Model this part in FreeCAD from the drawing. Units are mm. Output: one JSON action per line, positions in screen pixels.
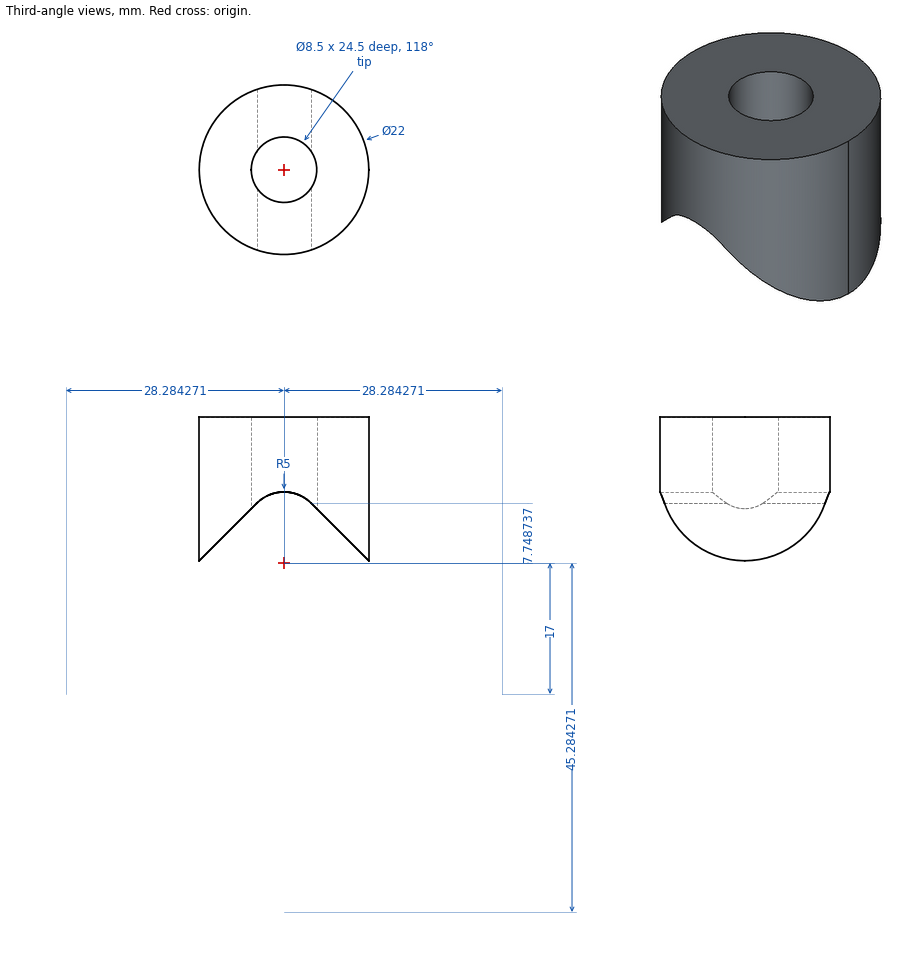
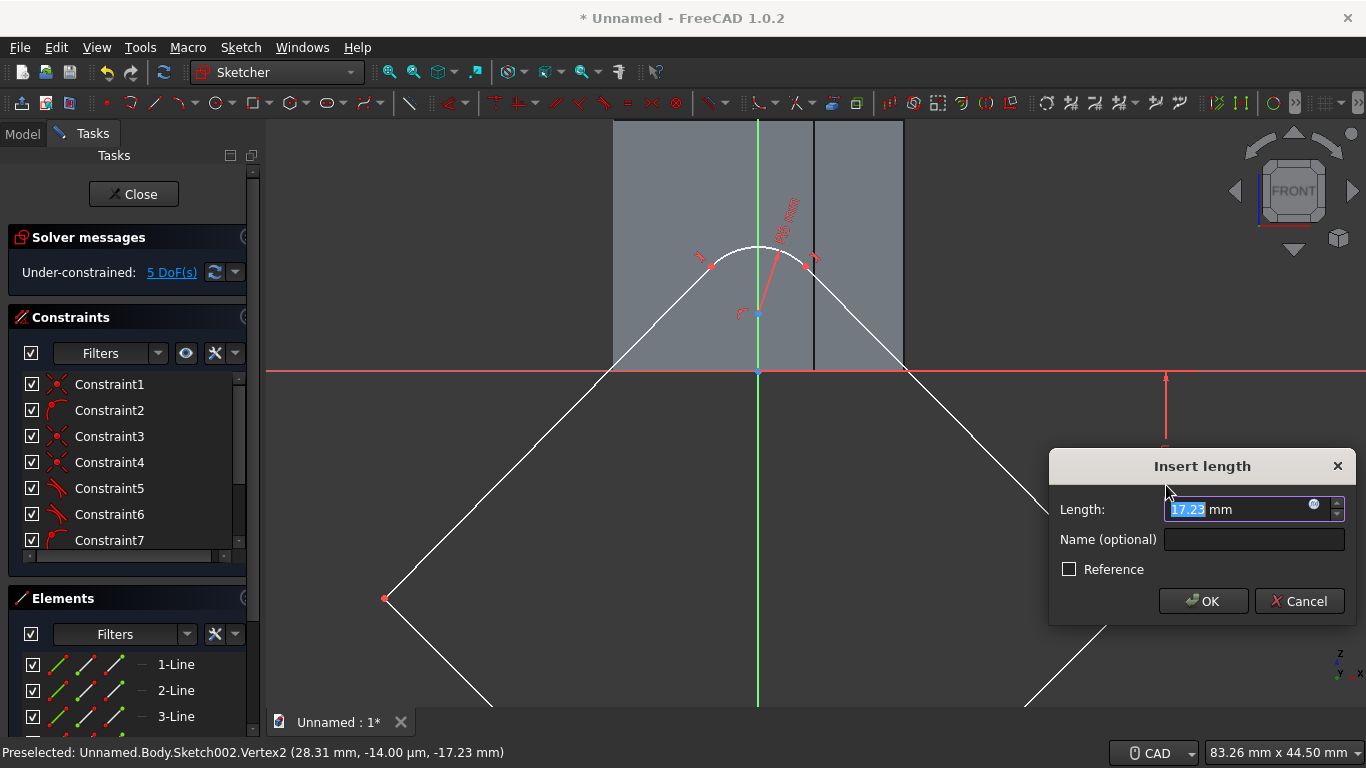
{"action": "type", "text": "17"}
{"action": "key", "text": "Return"}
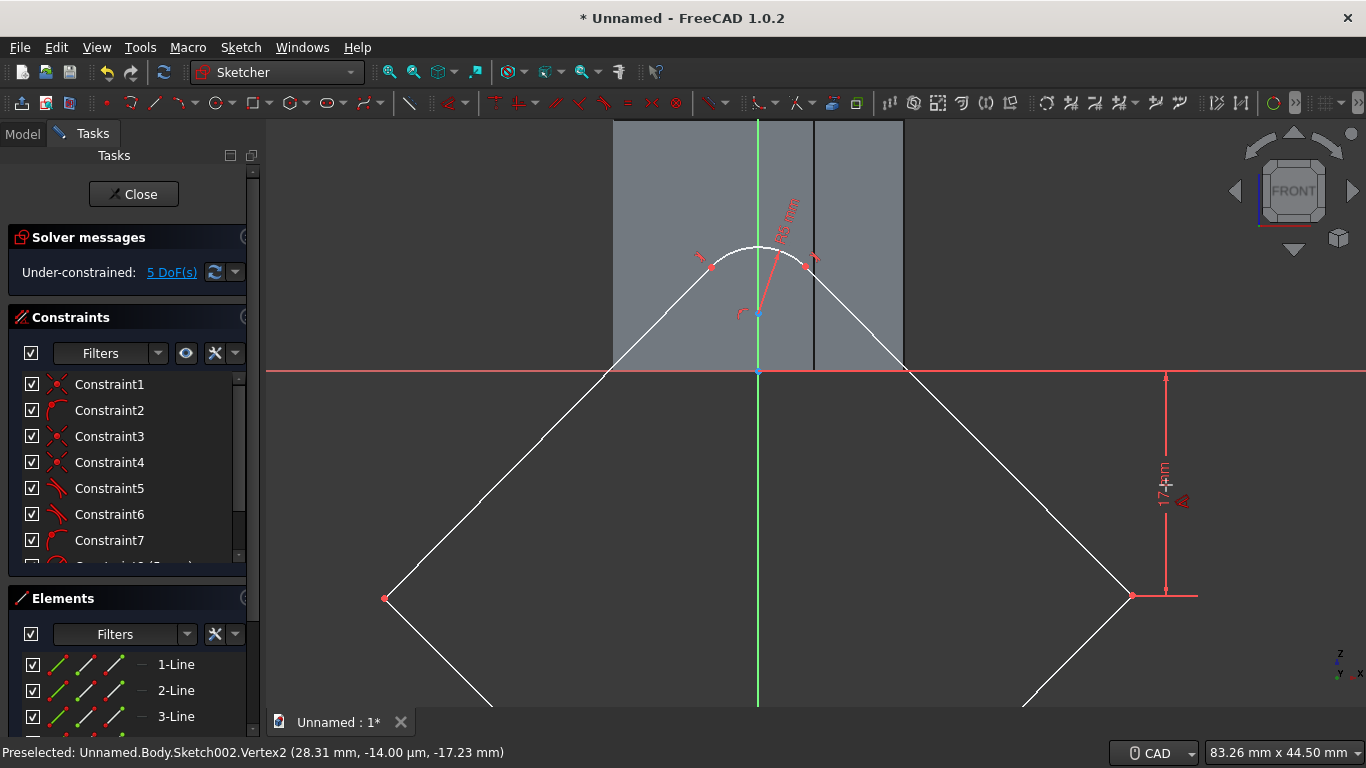
{"action": "left_click", "coordinate": [385, 599]}
{"action": "left_click", "coordinate": [351, 485]}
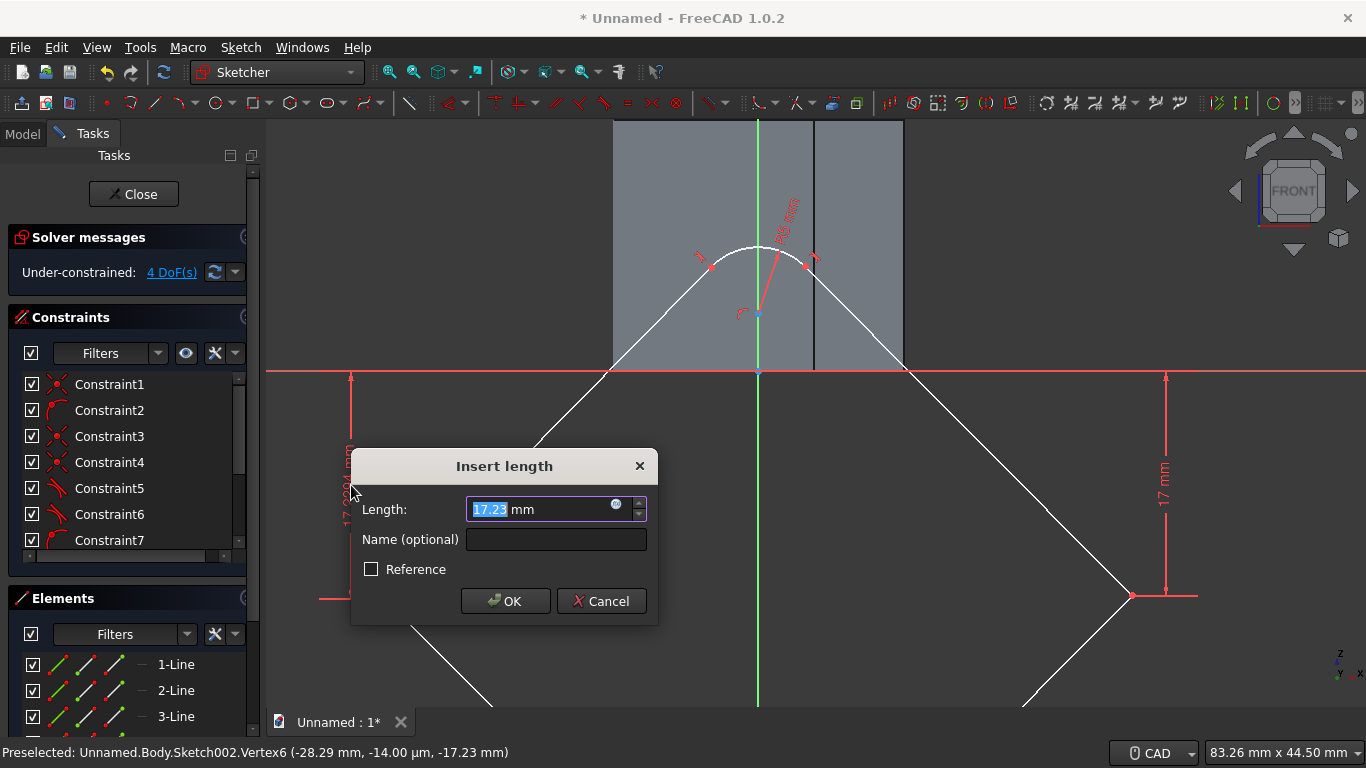
{"action": "type", "text": "17"}
{"action": "key", "text": "Return"}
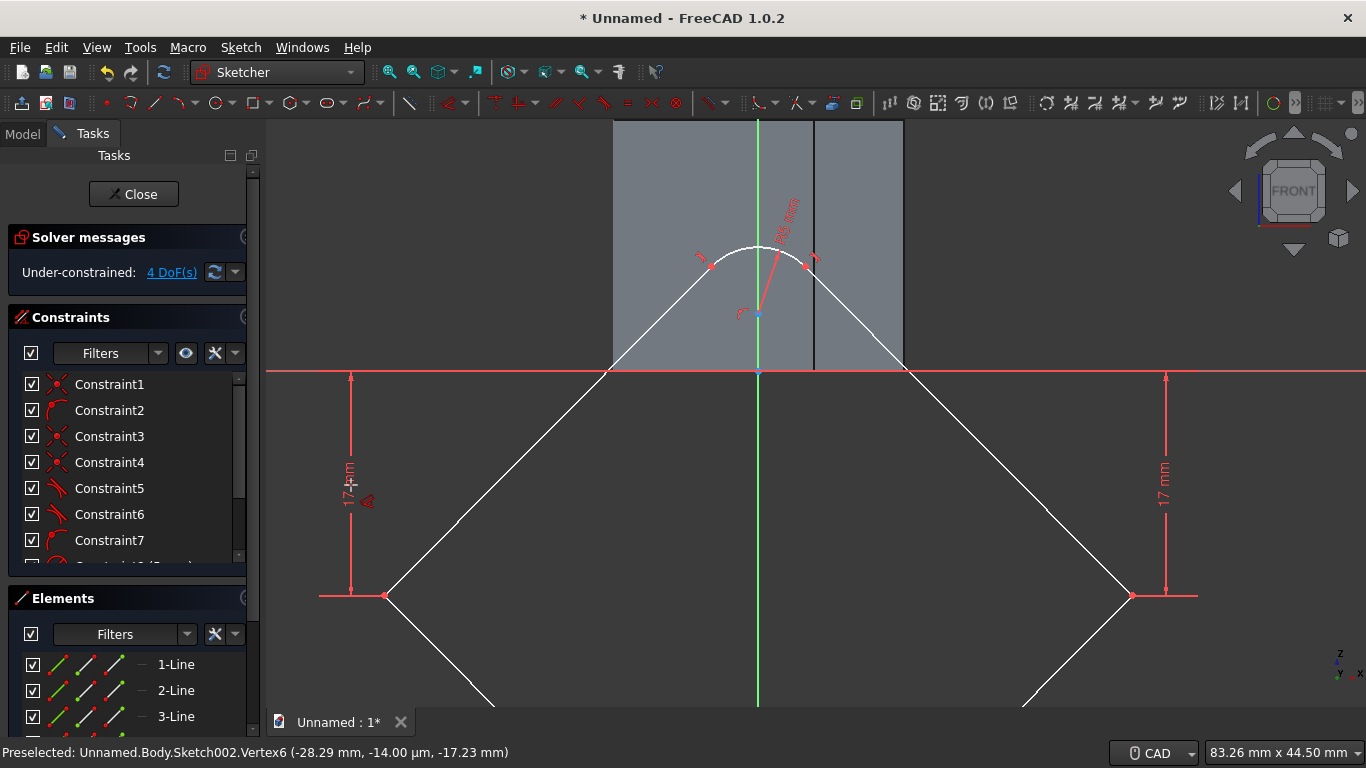
{"action": "left_click", "coordinate": [805, 267]}
{"action": "left_click", "coordinate": [839, 343]}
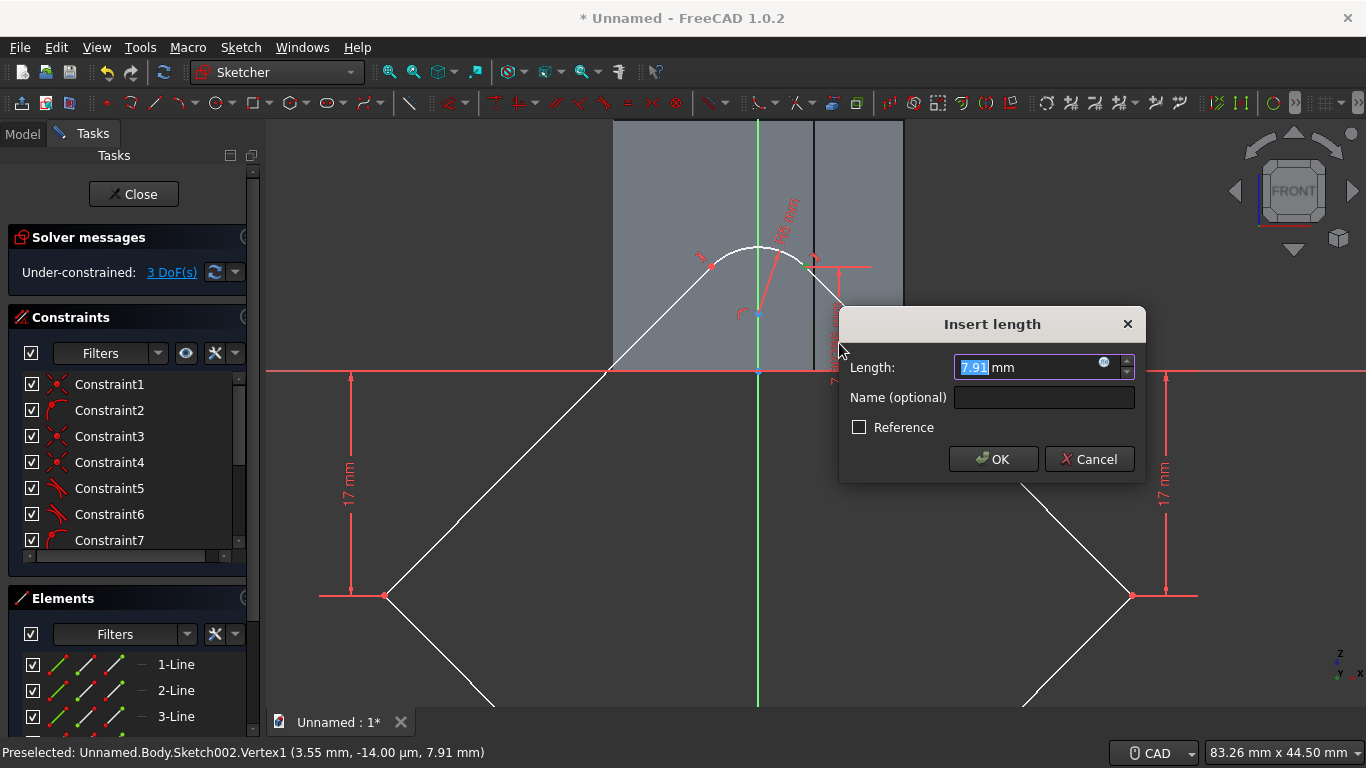
{"action": "type", "text": "7.748737"}
{"action": "key", "text": "Return"}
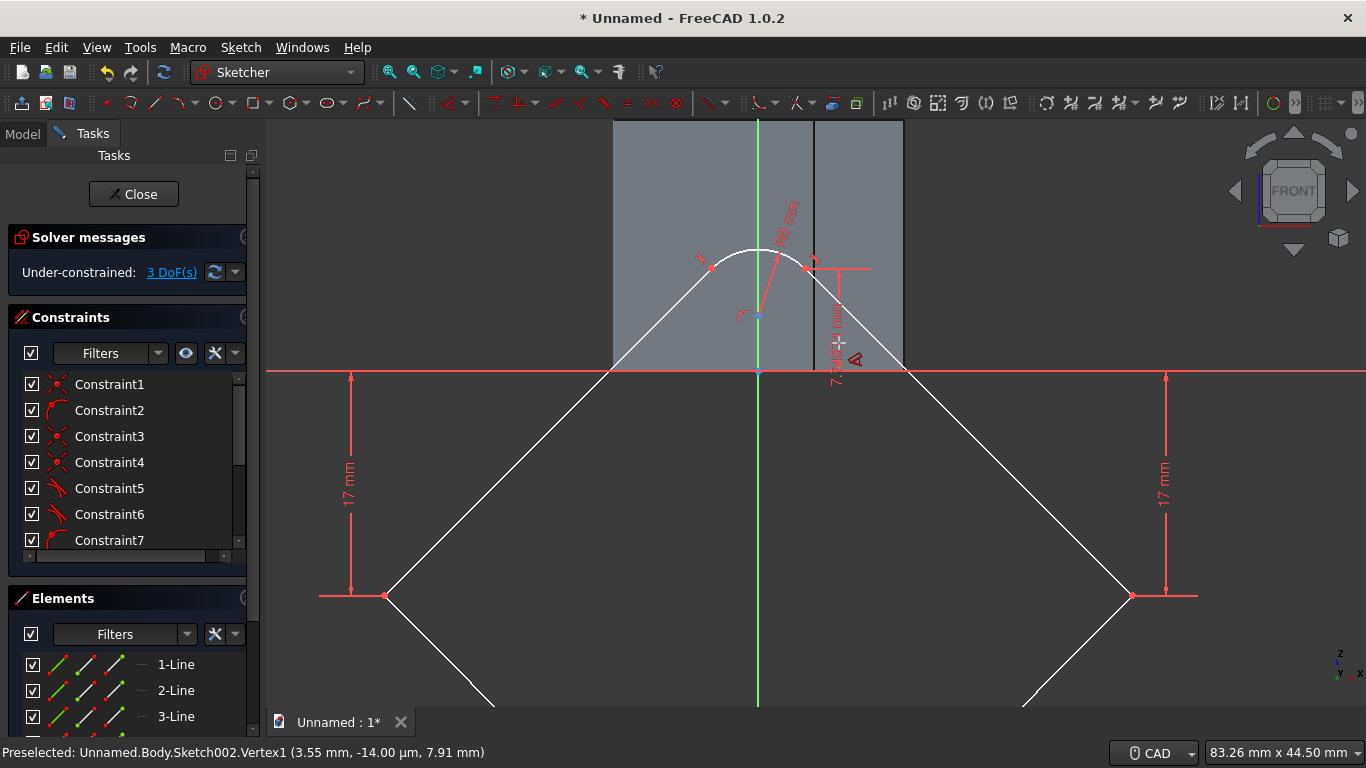
{"action": "left_click", "coordinate": [1132, 596]}
{"action": "left_click", "coordinate": [945, 337]}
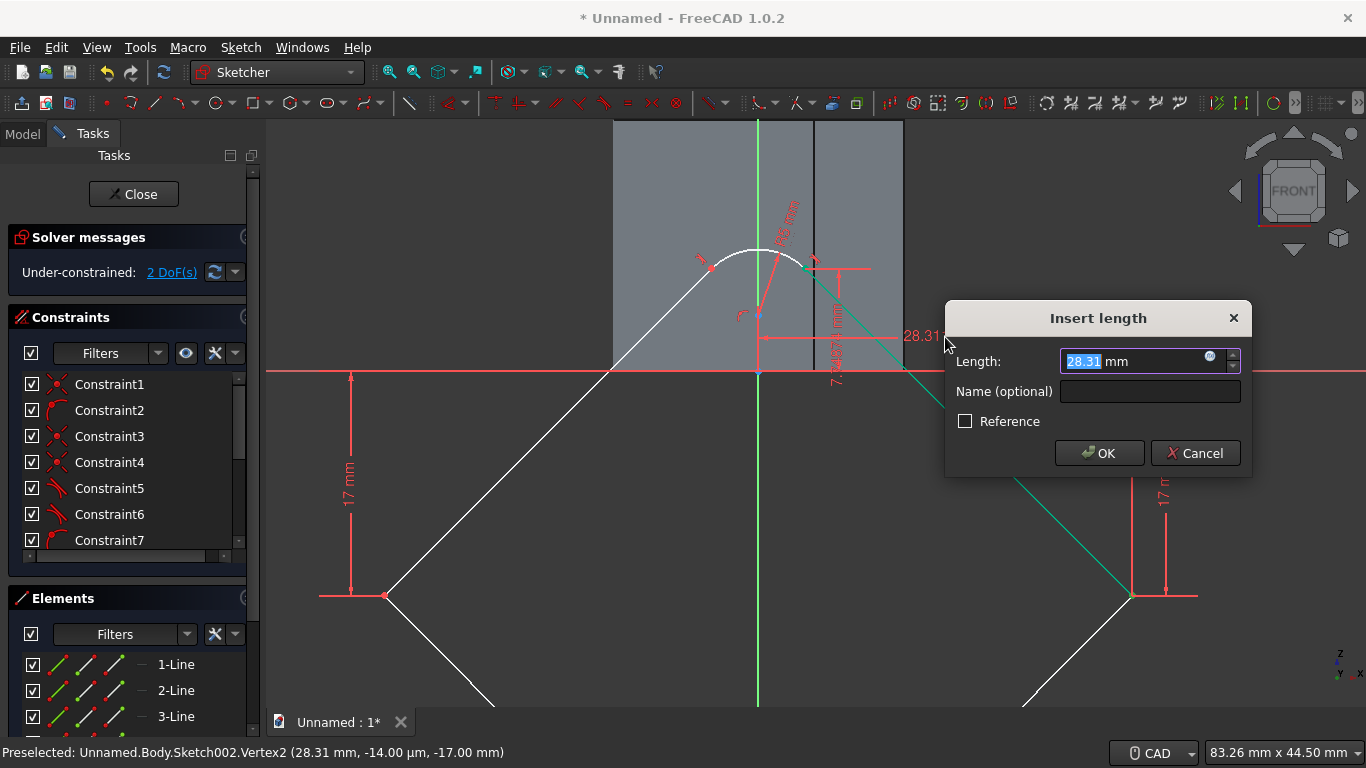
{"action": "type", "text": "28.284271"}
{"action": "key", "text": "Return"}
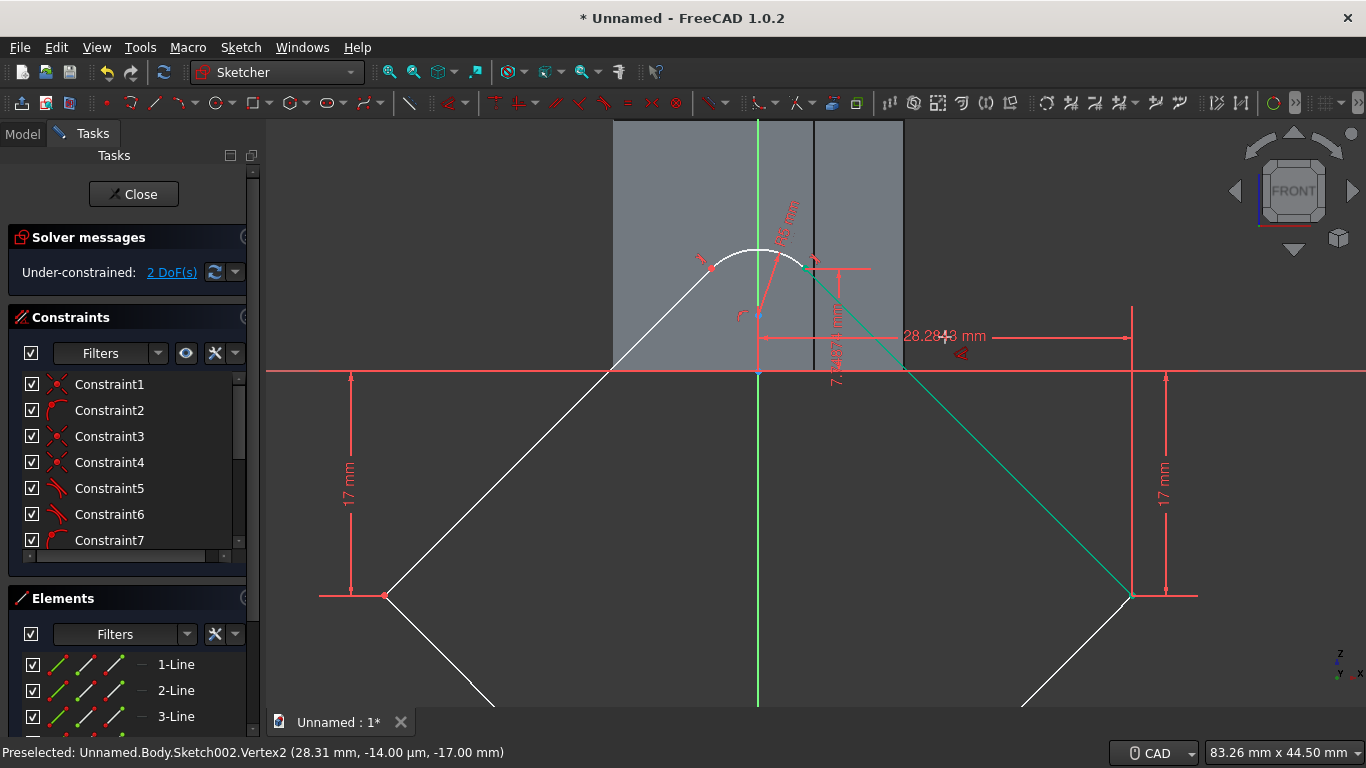
{"action": "scroll", "coordinate": [734, 174], "scroll_direction": "down", "scroll_amount": 3}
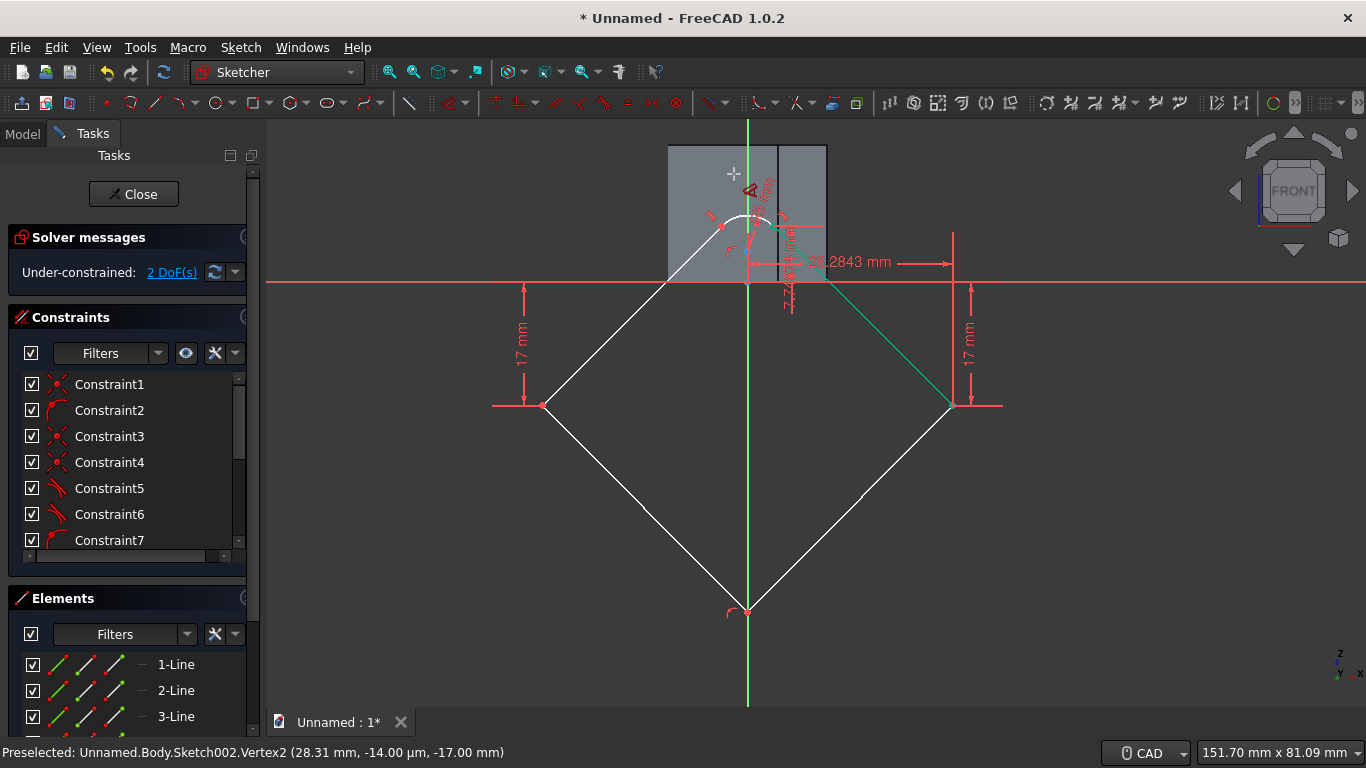
{"action": "left_click", "coordinate": [748, 612]}
{"action": "left_click", "coordinate": [782, 447]}